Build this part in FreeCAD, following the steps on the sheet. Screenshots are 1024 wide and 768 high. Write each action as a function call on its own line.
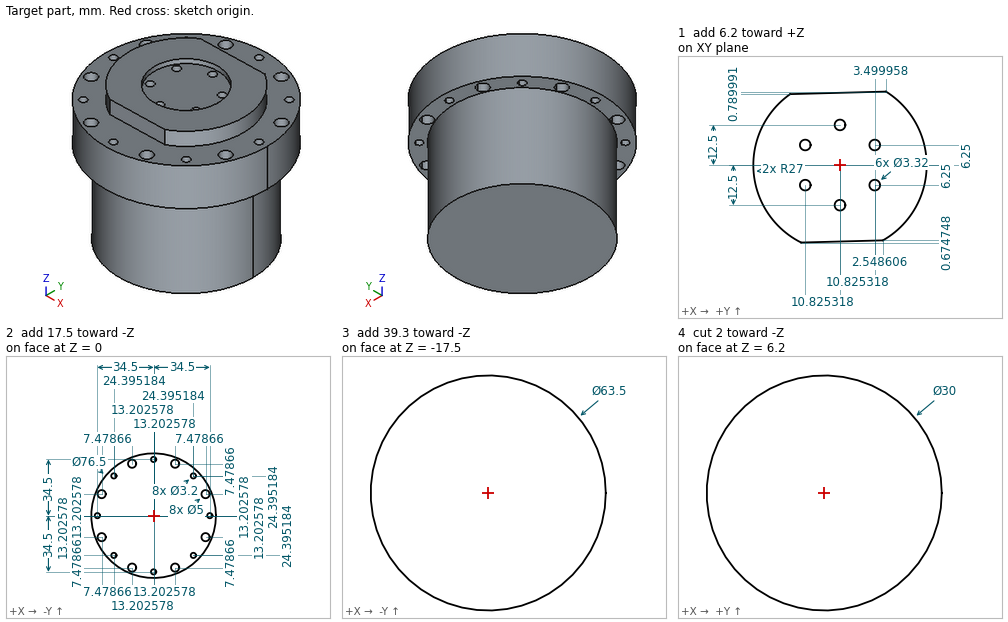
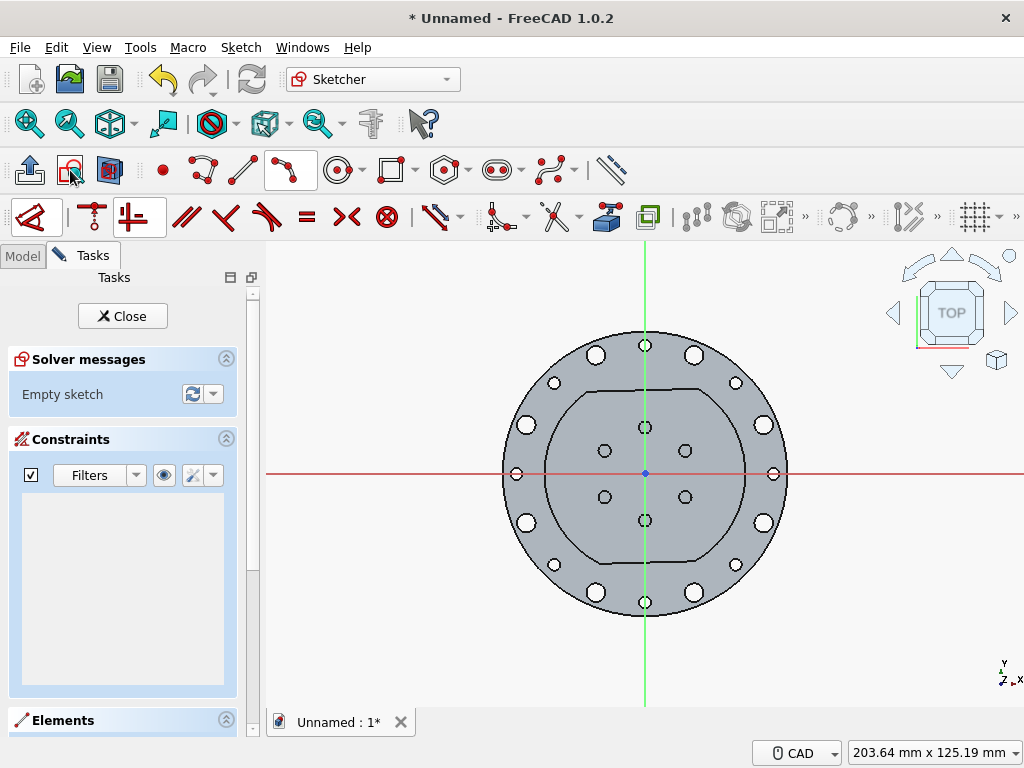
scroll(685, 474, up, 5)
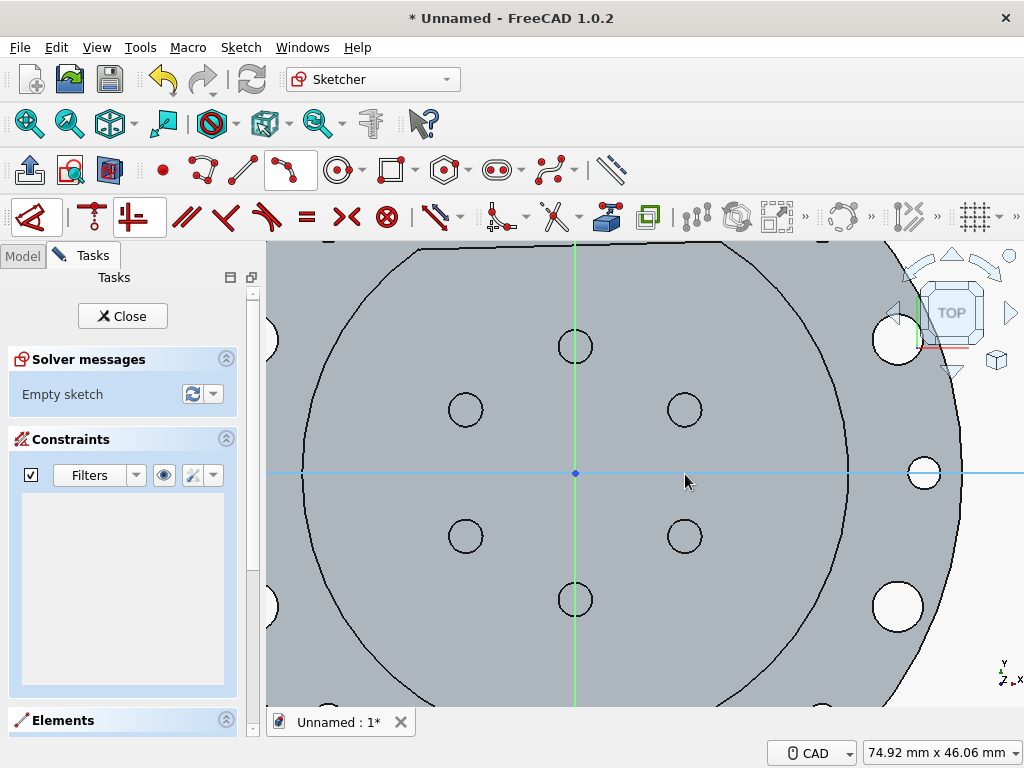
click(338, 170)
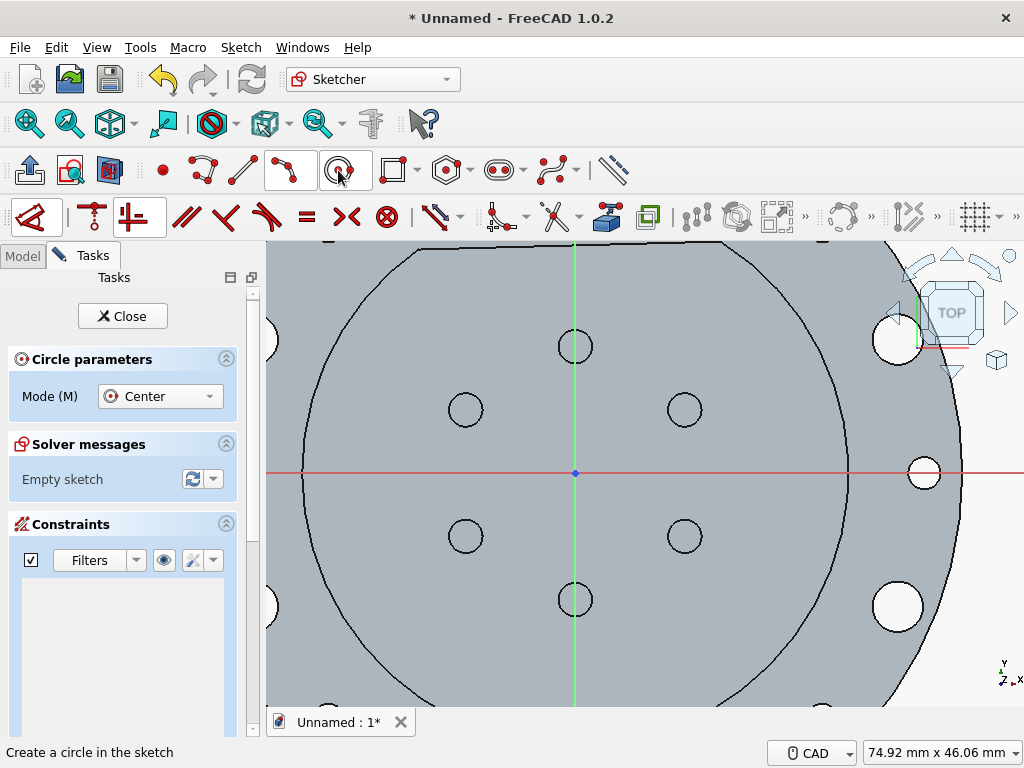
click(575, 473)
move(683, 366)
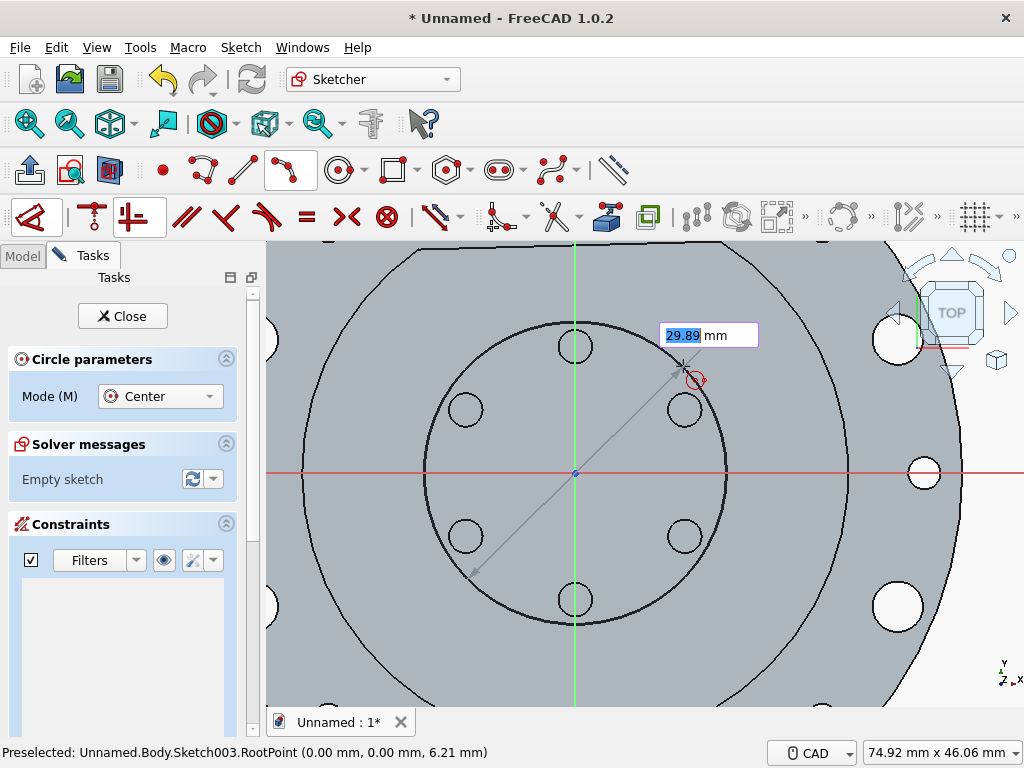
text(30)
key(Return)
key(Escape)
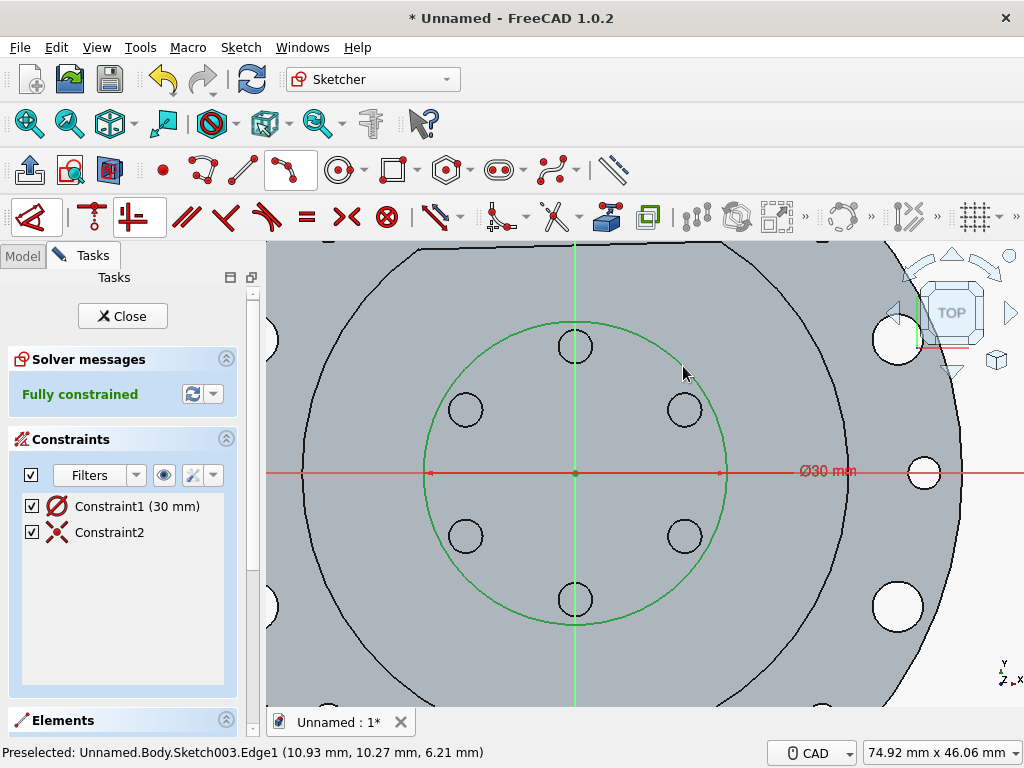
click(123, 316)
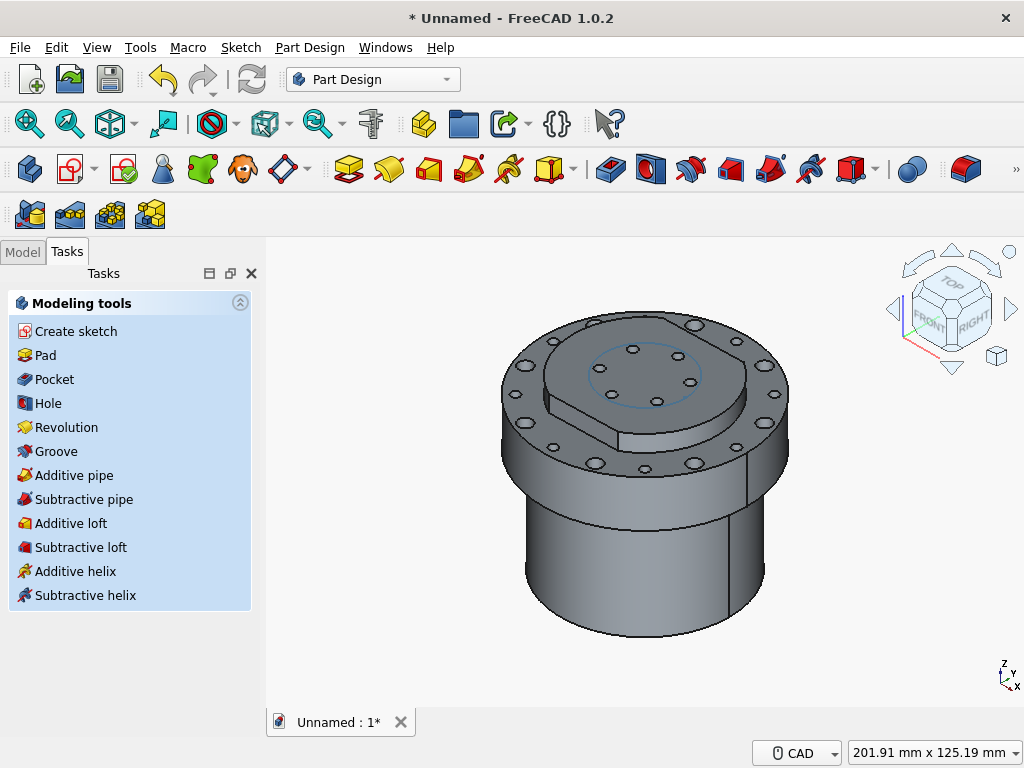
click(612, 170)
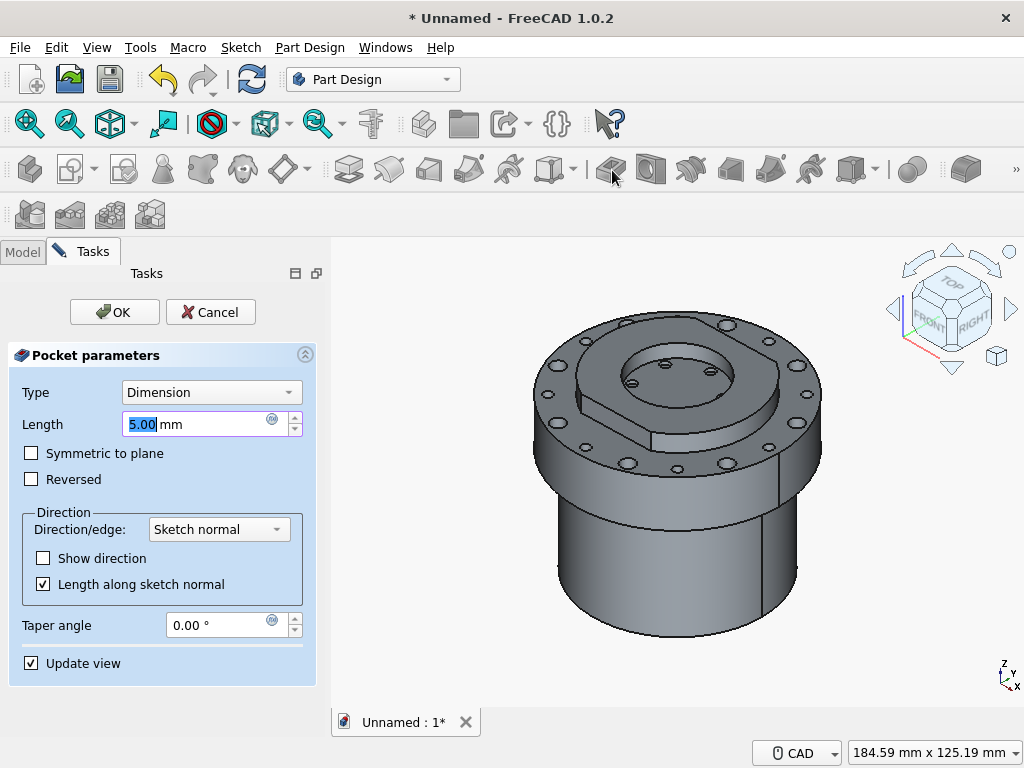
text(2)
key(Tab)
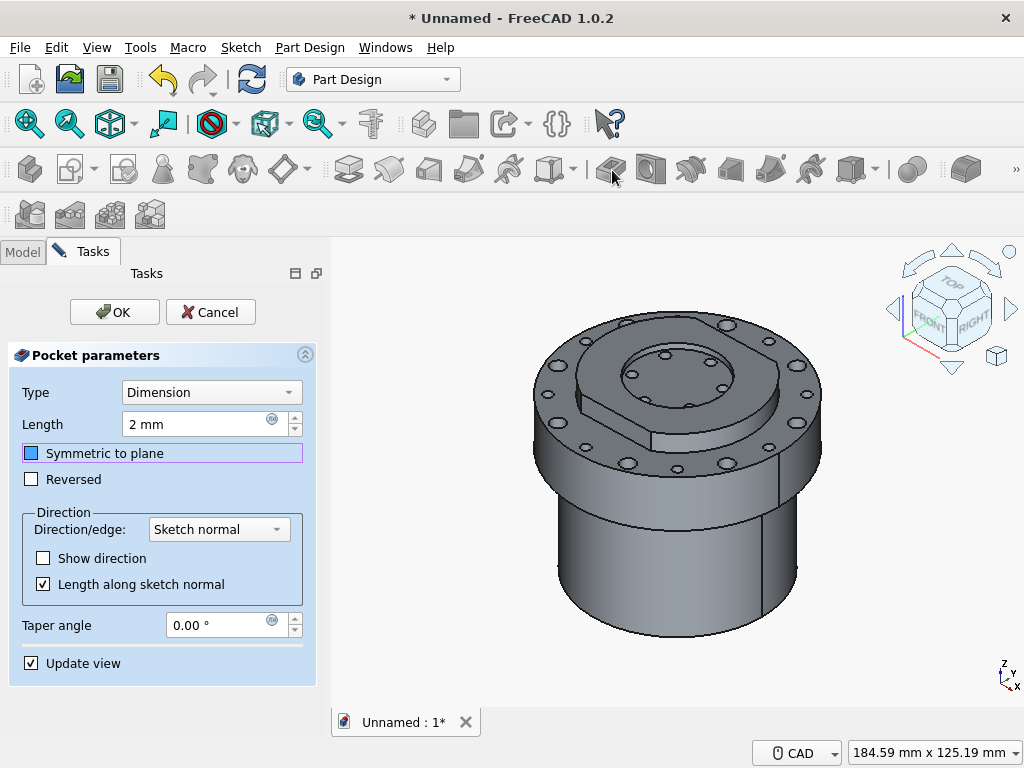
click(115, 312)